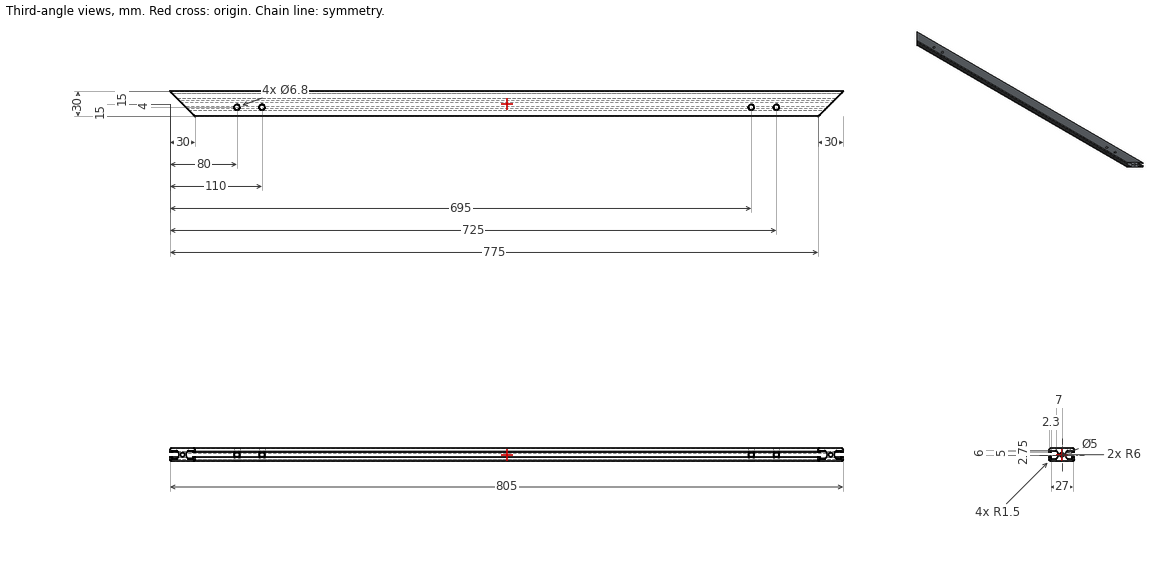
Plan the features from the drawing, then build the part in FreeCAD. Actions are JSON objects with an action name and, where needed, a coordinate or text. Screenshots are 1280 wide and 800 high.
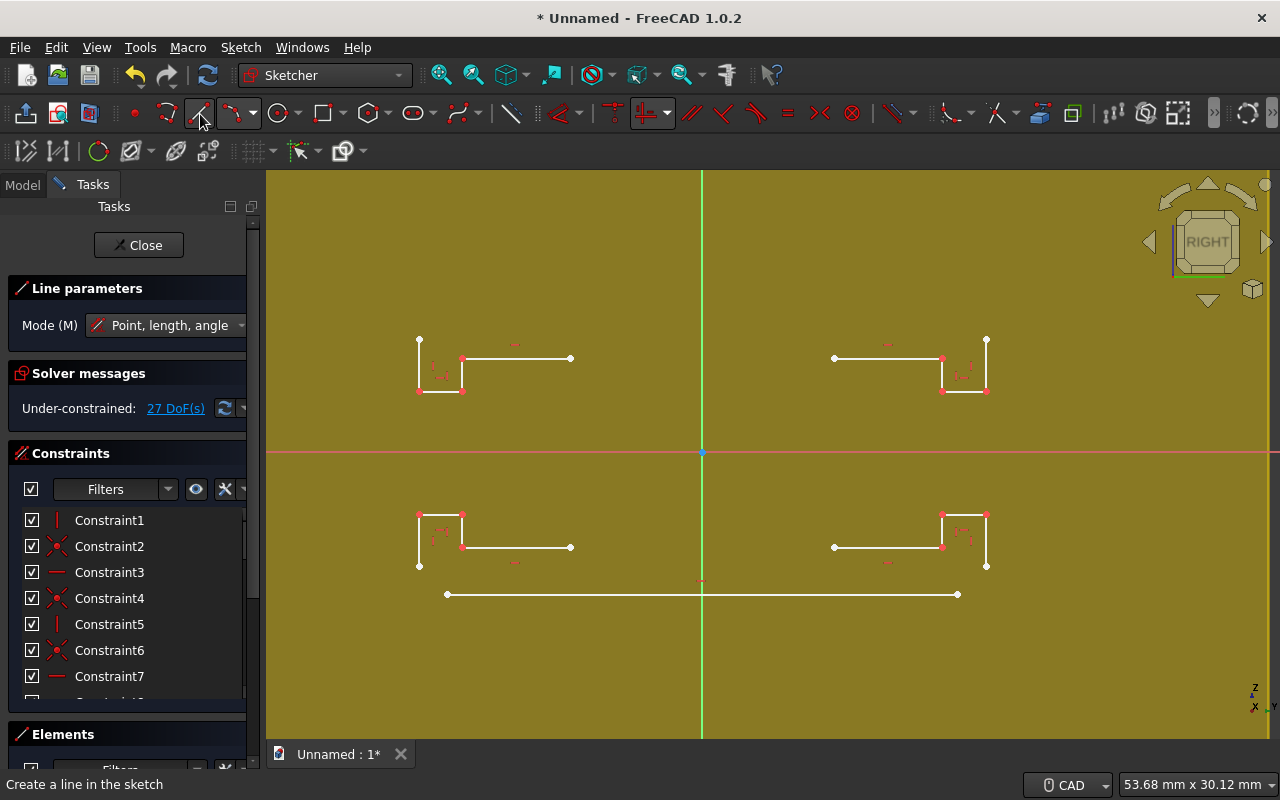
{"action": "left_click", "coordinate": [957, 310]}
{"action": "left_click", "coordinate": [447, 310]}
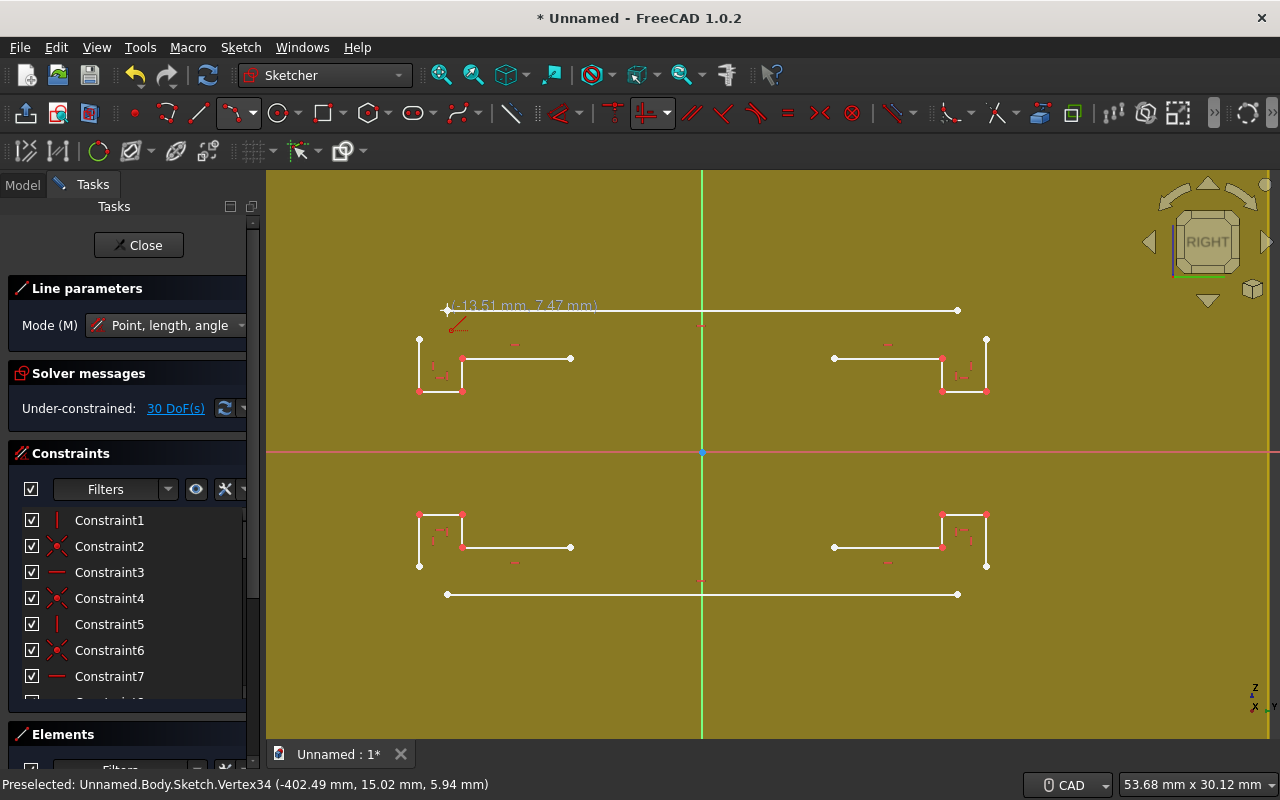
{"action": "left_click", "coordinate": [232, 114]}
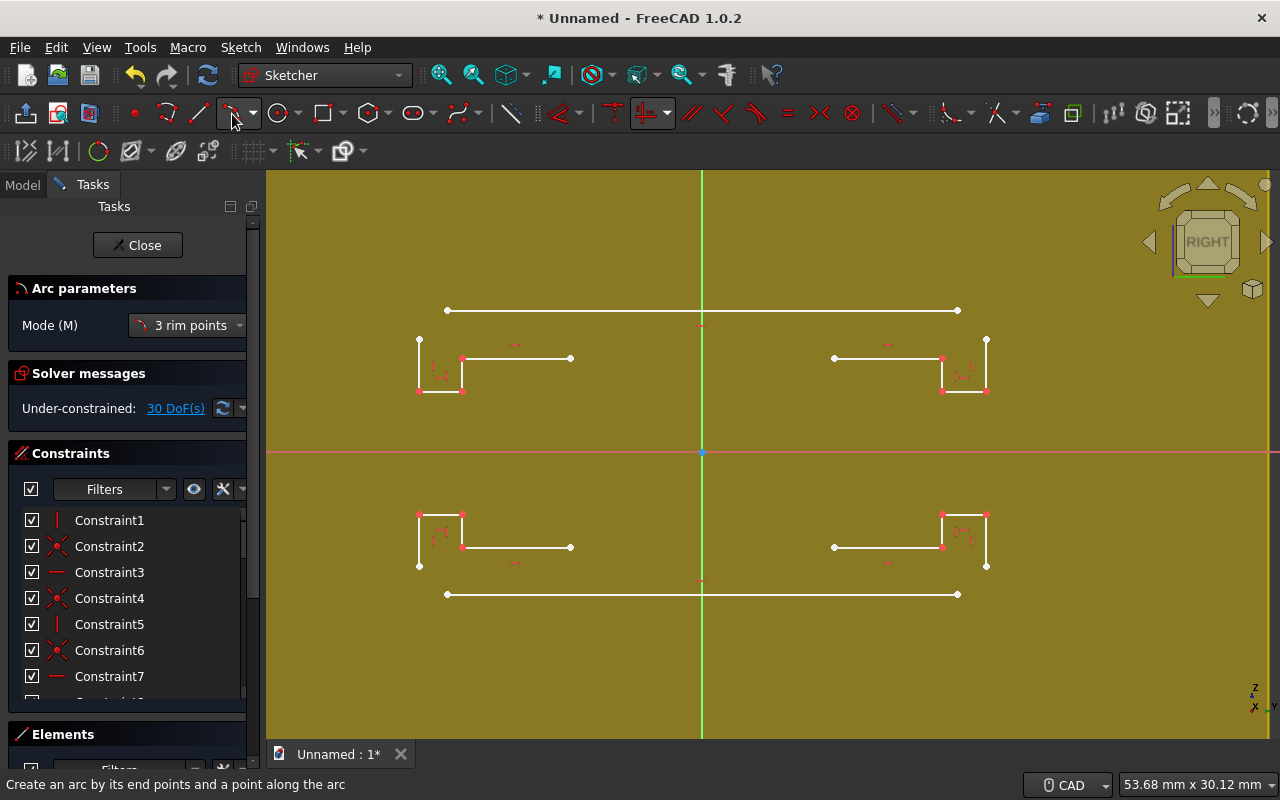
{"action": "left_click", "coordinate": [570, 359]}
{"action": "left_click", "coordinate": [570, 548]}
{"action": "left_click", "coordinate": [618, 474]}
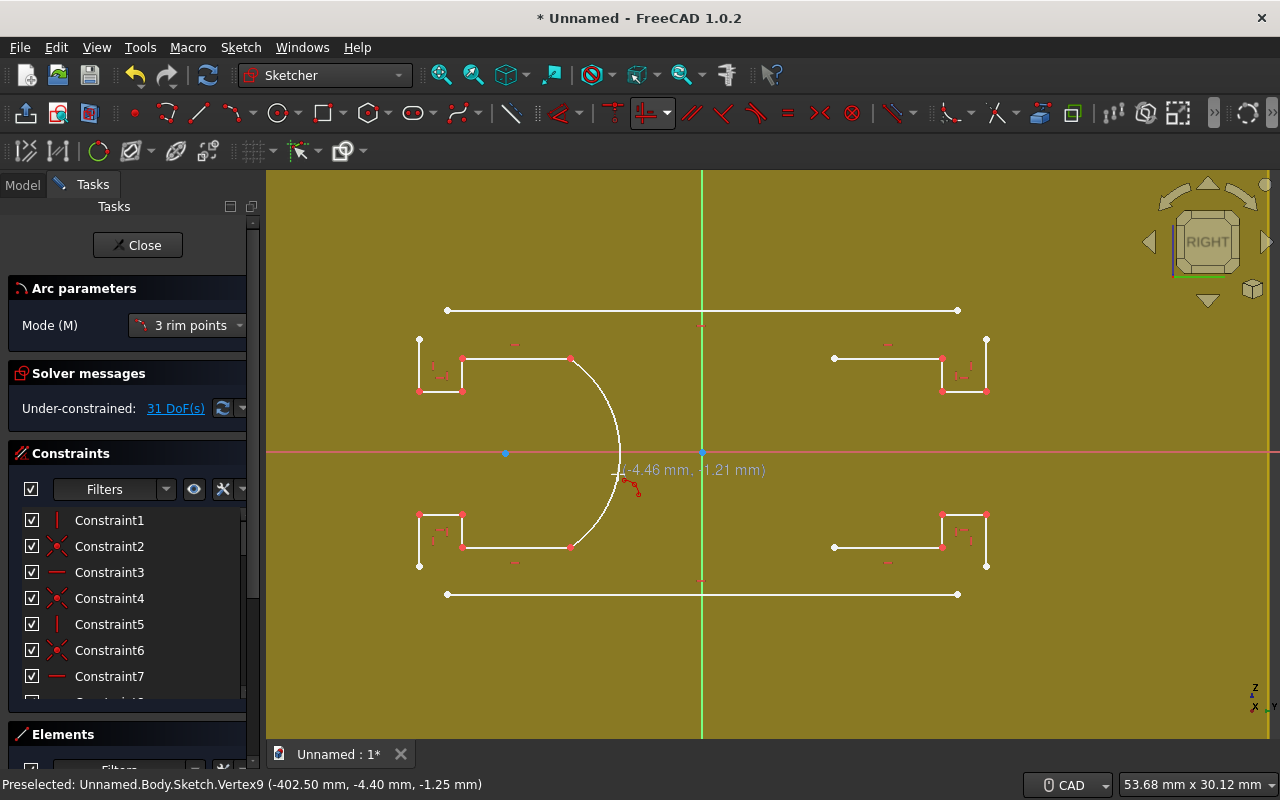
{"action": "left_click", "coordinate": [419, 567]}
{"action": "left_click", "coordinate": [447, 595]}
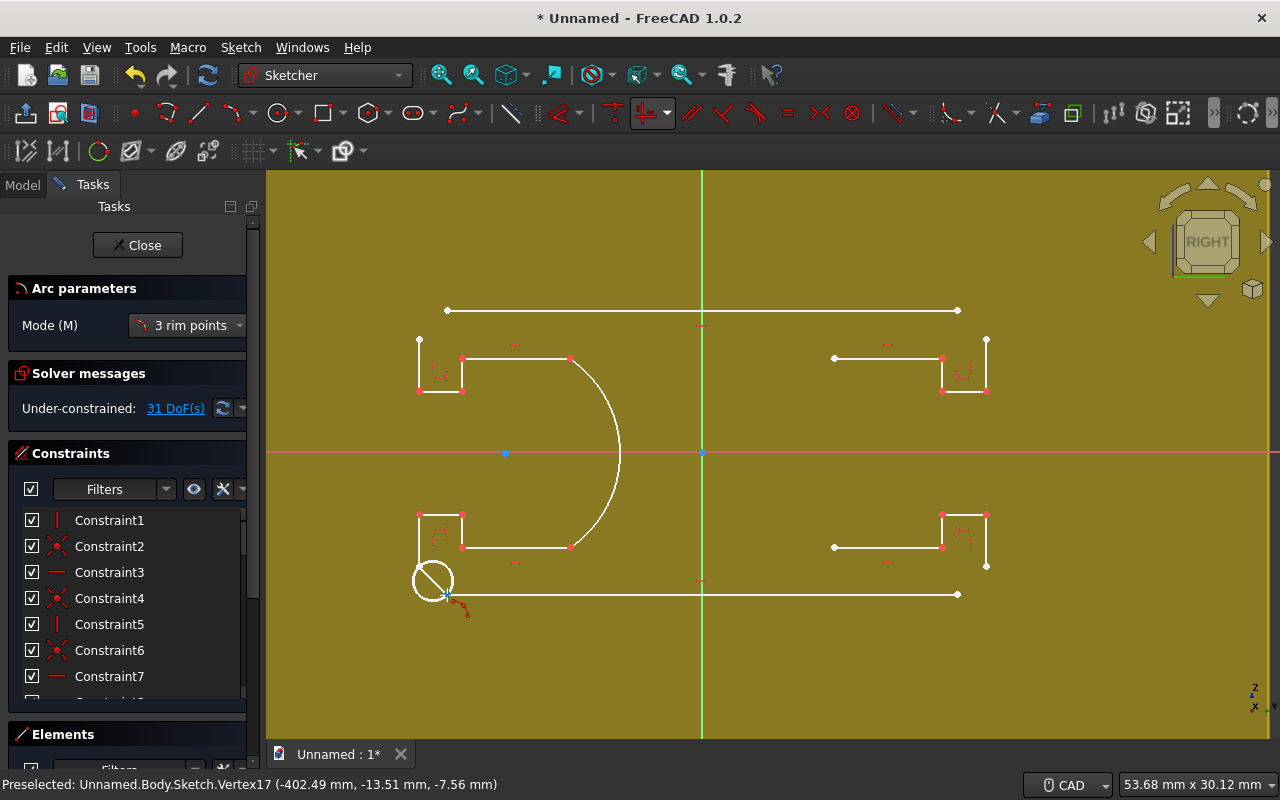
{"action": "scroll", "coordinate": [427, 586], "scroll_direction": "up", "scroll_amount": 4}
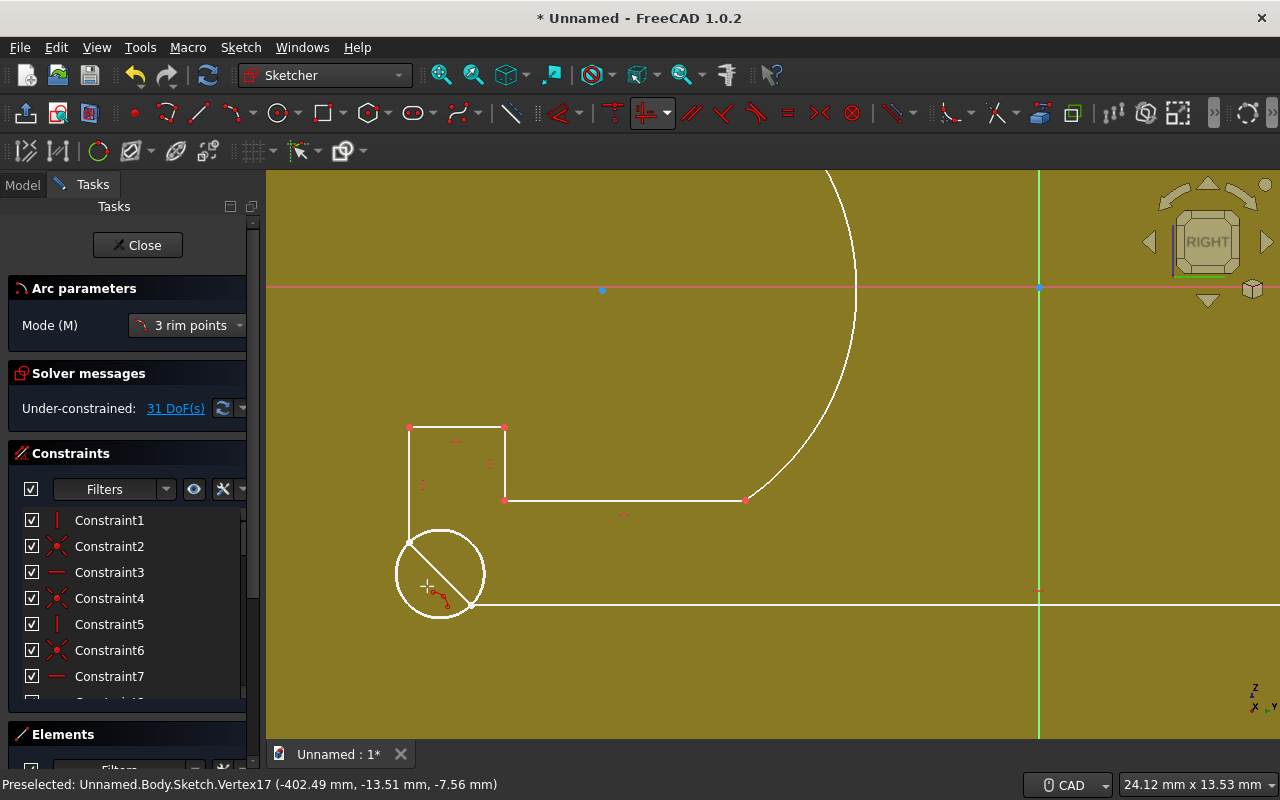
{"action": "left_click", "coordinate": [427, 584]}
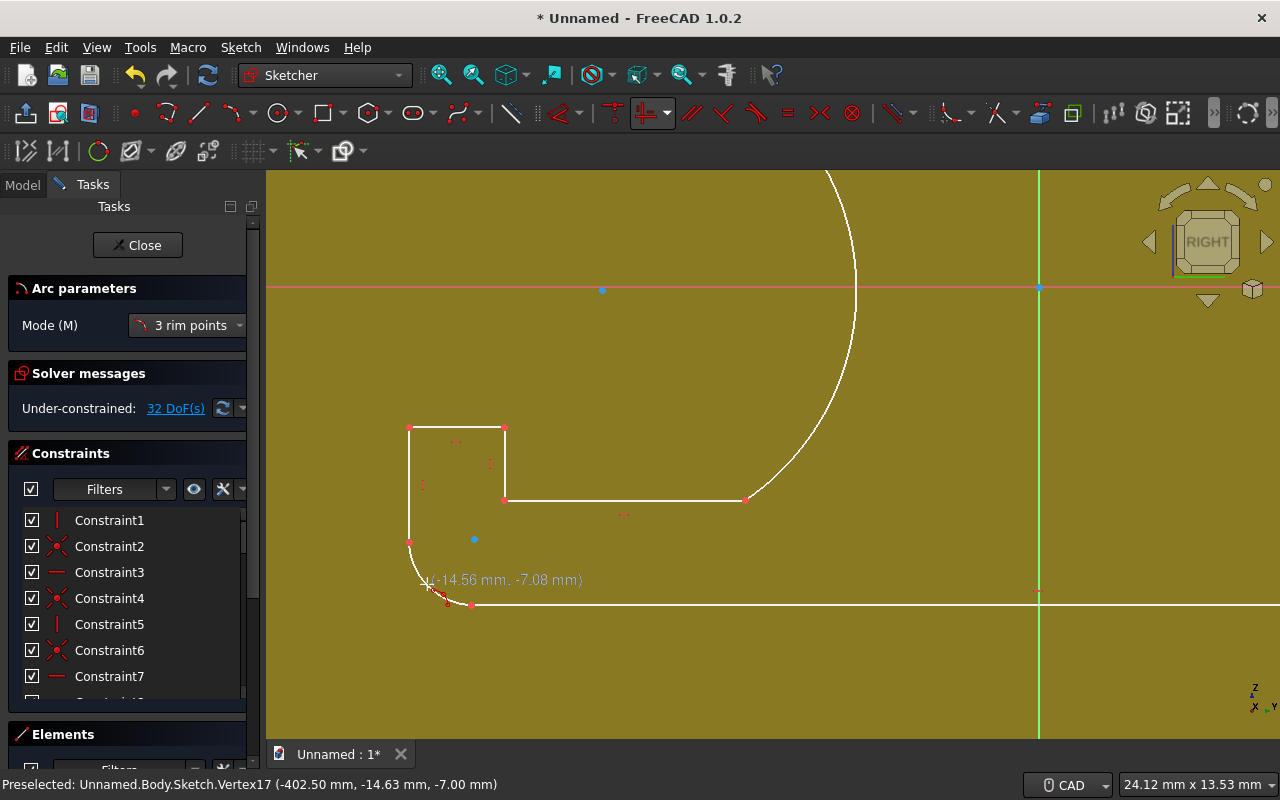
{"action": "scroll", "coordinate": [431, 591], "scroll_direction": "down", "scroll_amount": 4}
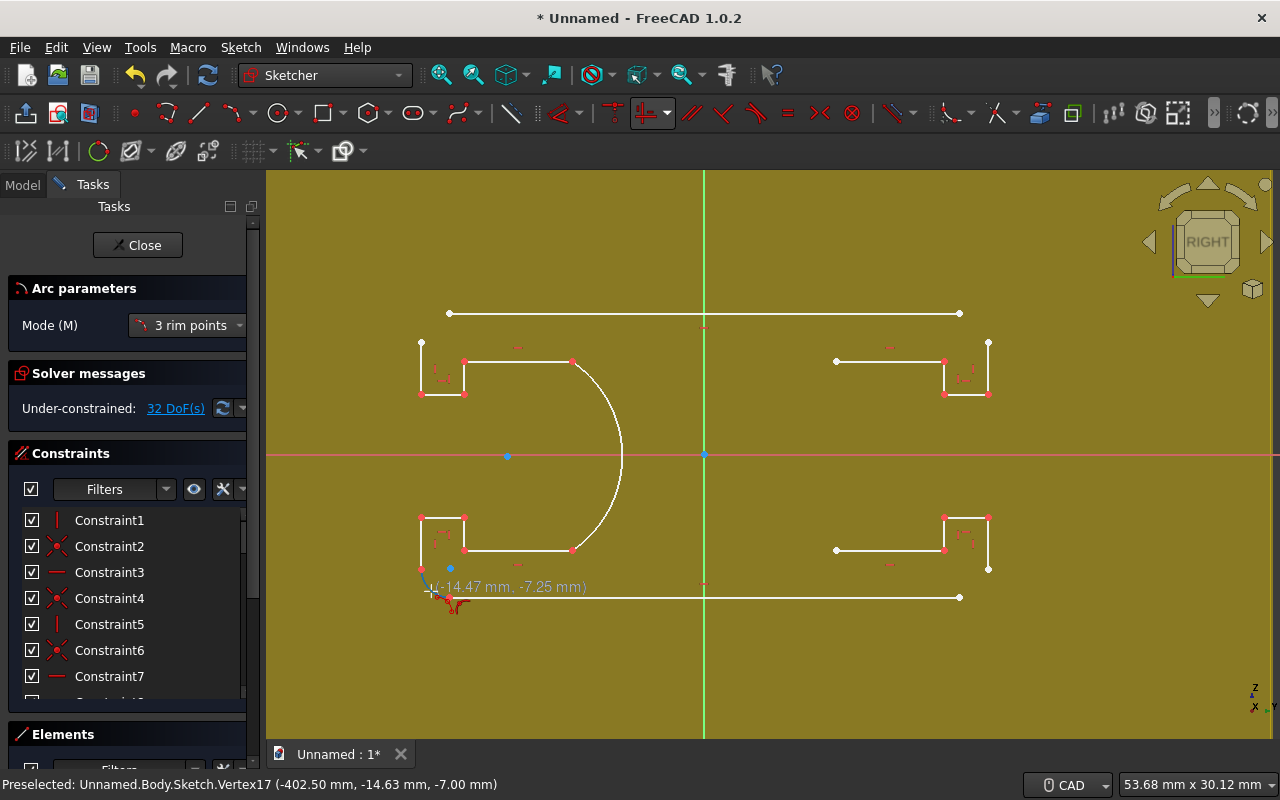
{"action": "left_click", "coordinate": [959, 598]}
{"action": "left_click", "coordinate": [988, 570]}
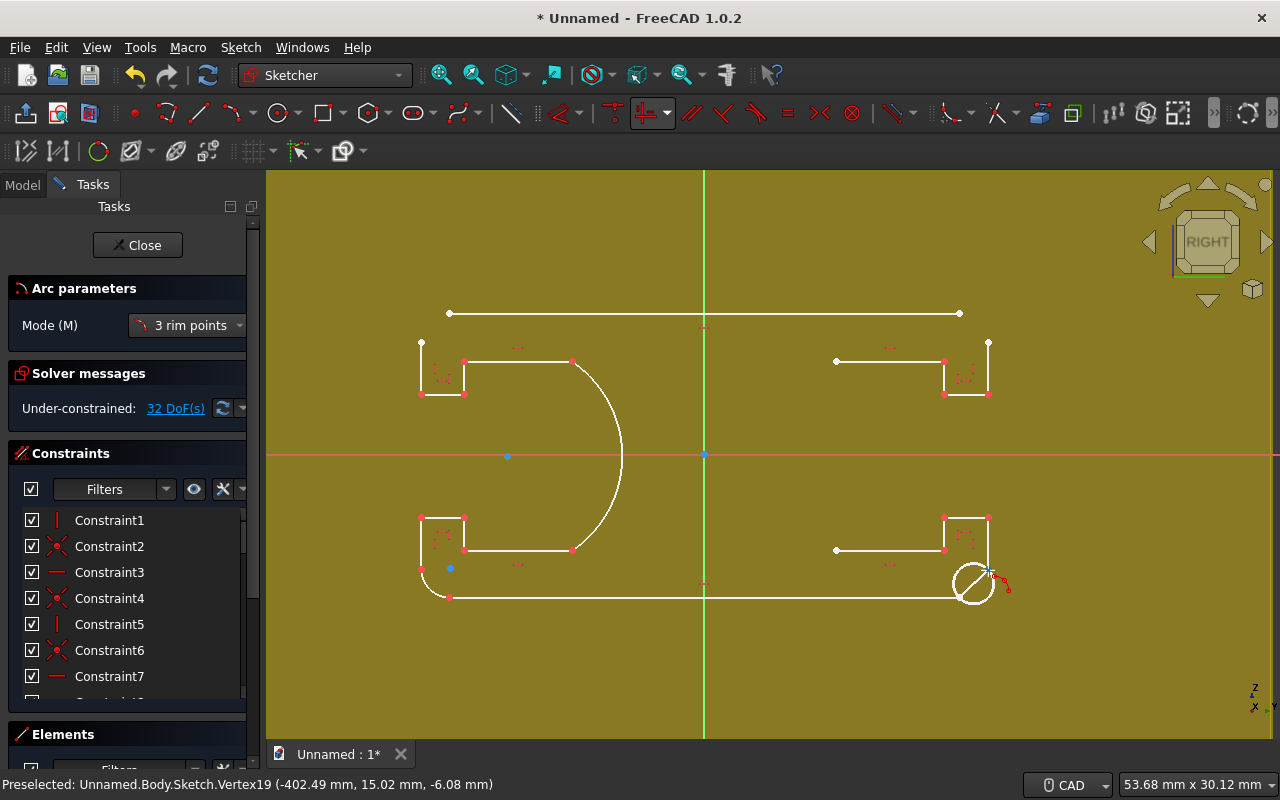
{"action": "scroll", "coordinate": [979, 588], "scroll_direction": "up", "scroll_amount": 4}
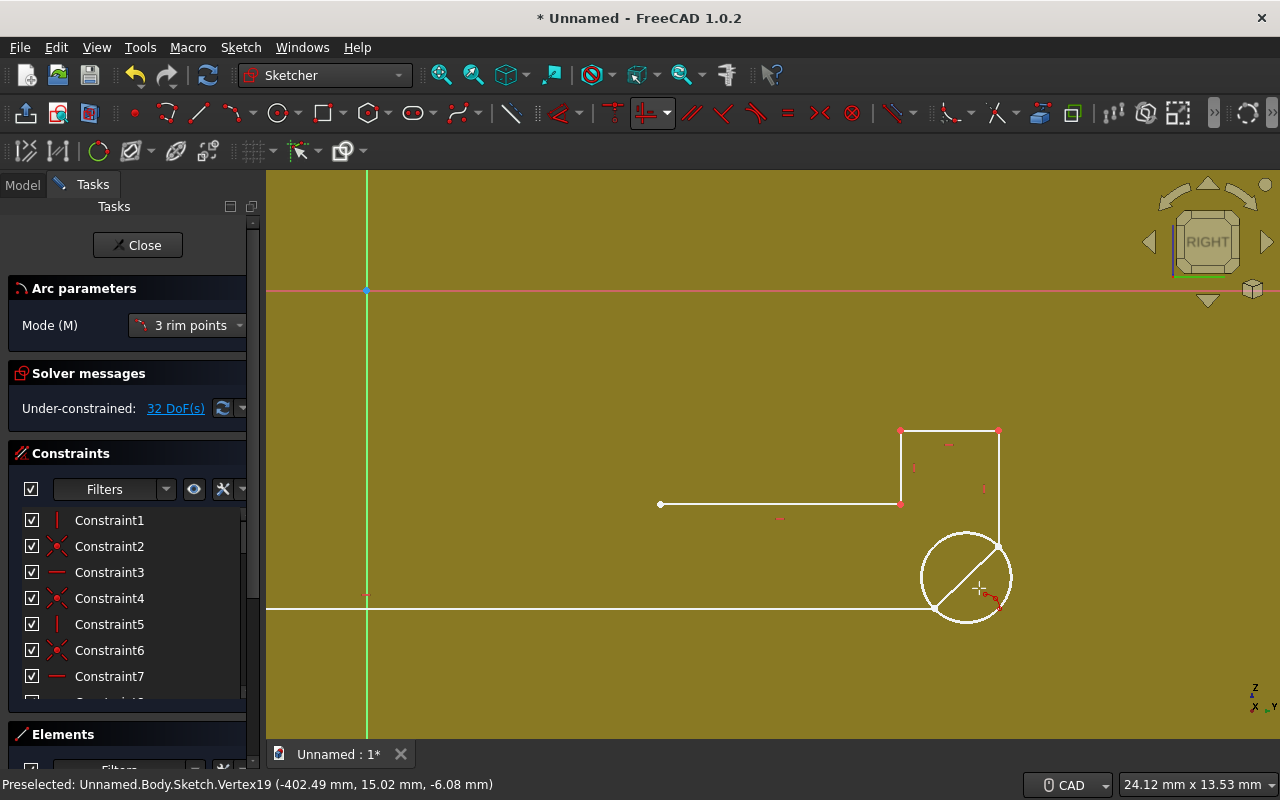
{"action": "left_click", "coordinate": [979, 588]}